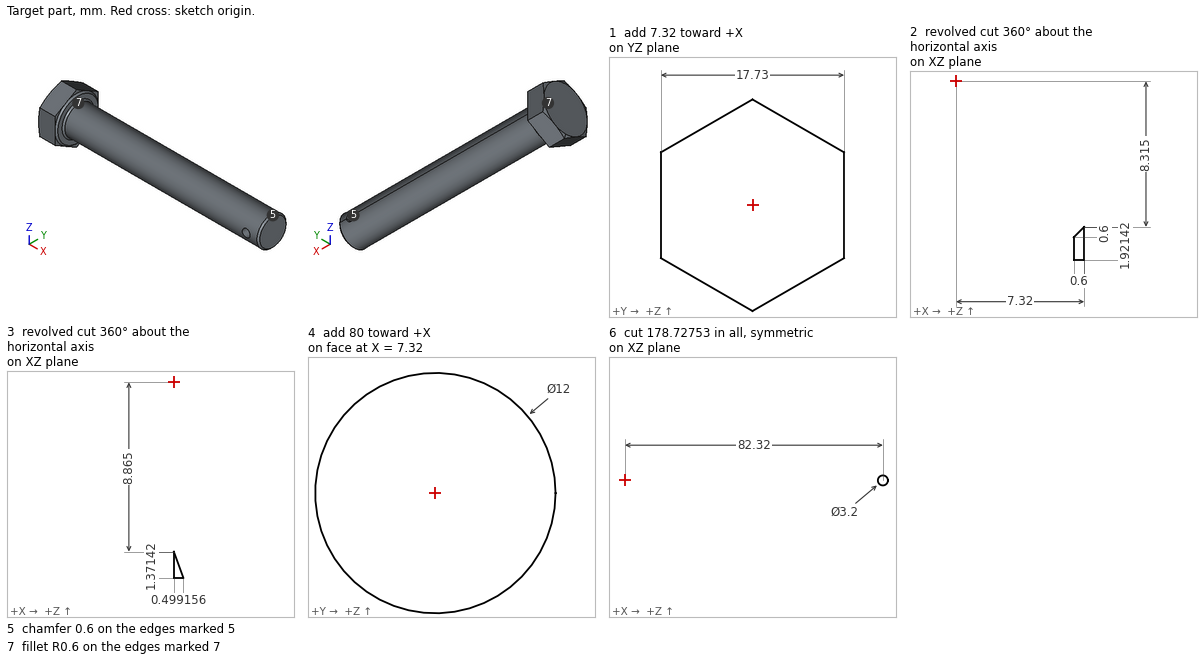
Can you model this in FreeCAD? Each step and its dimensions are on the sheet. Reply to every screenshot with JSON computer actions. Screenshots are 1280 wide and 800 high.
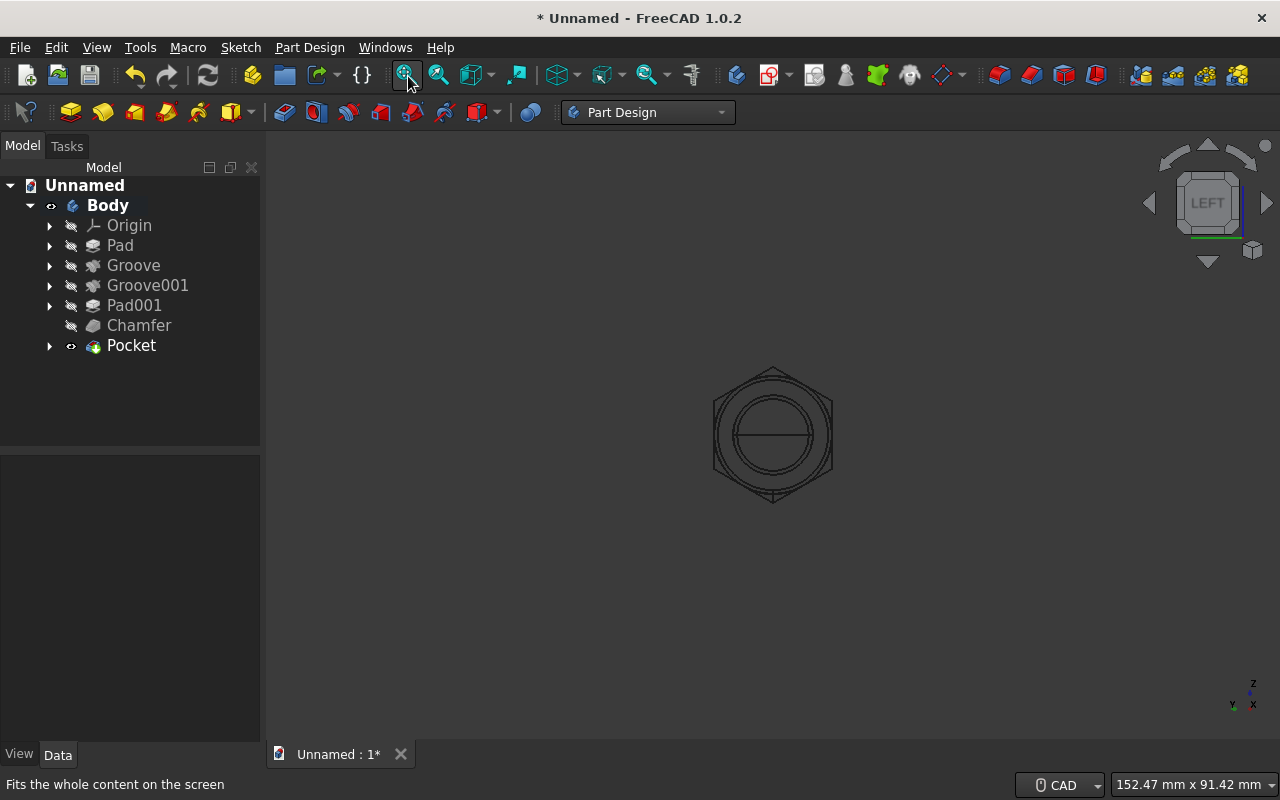
{"action": "key", "text": "0"}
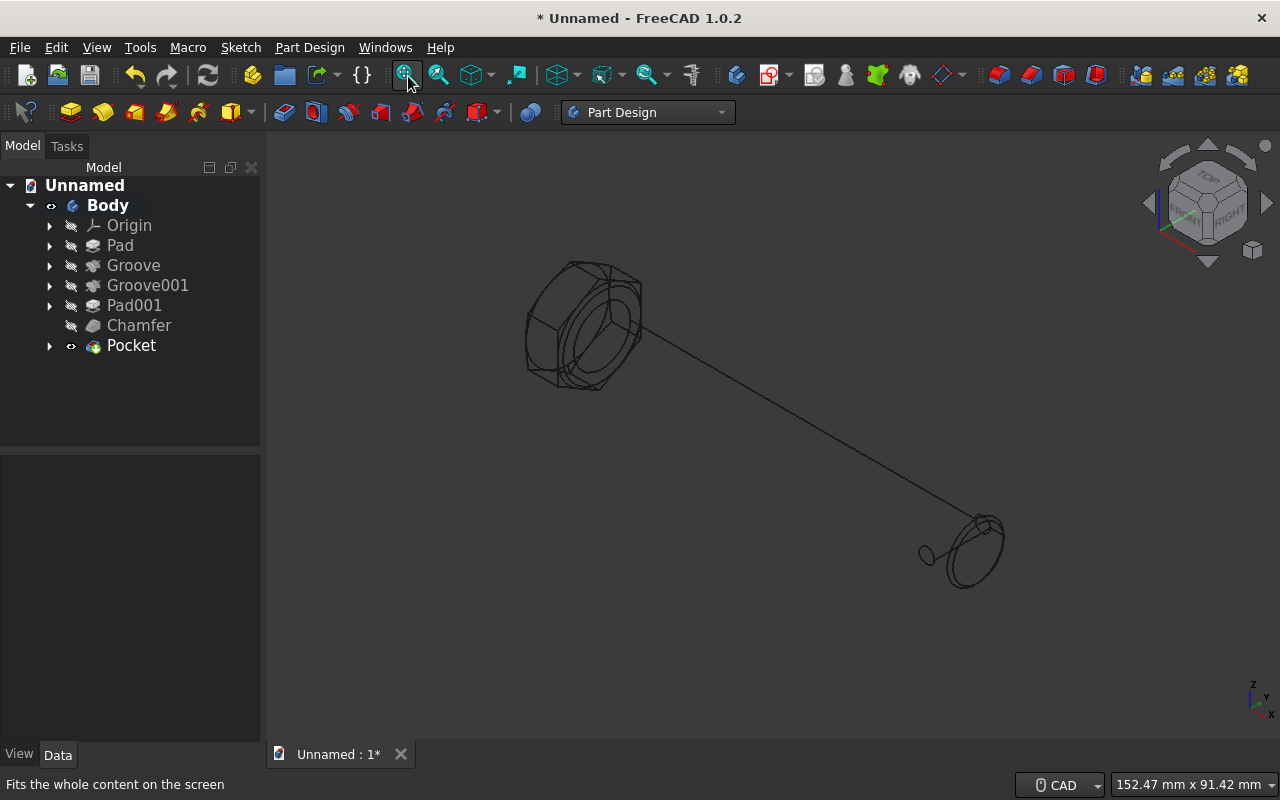
{"action": "left_click", "coordinate": [574, 352]}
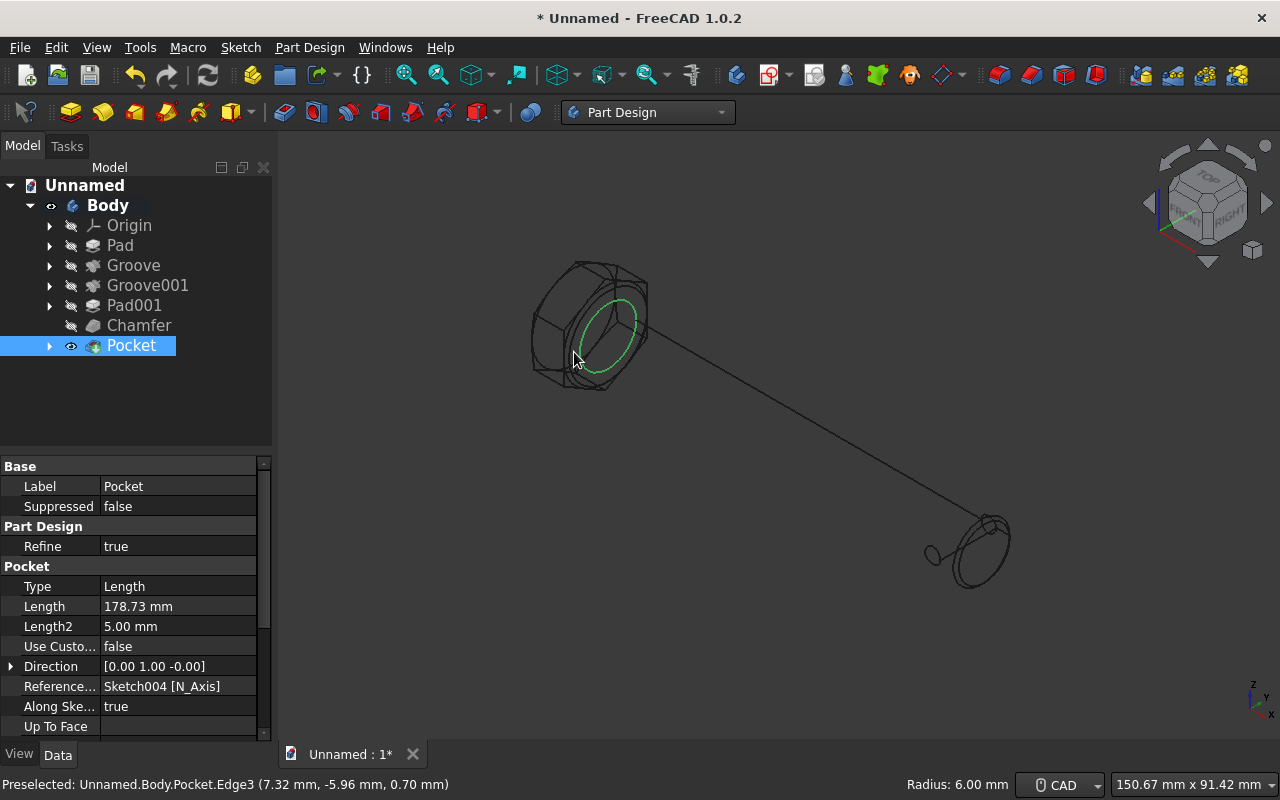
{"action": "key", "text": "v 1"}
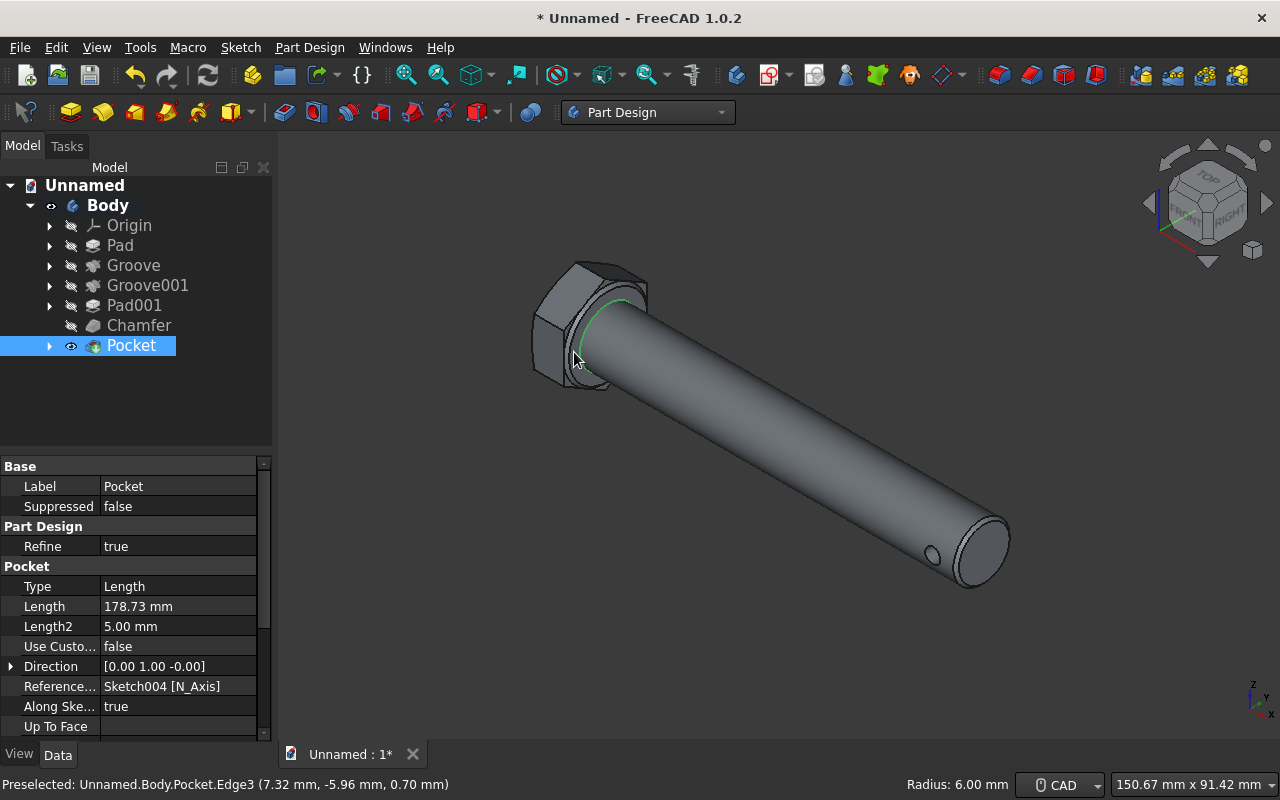
{"action": "left_click", "coordinate": [1000, 76]}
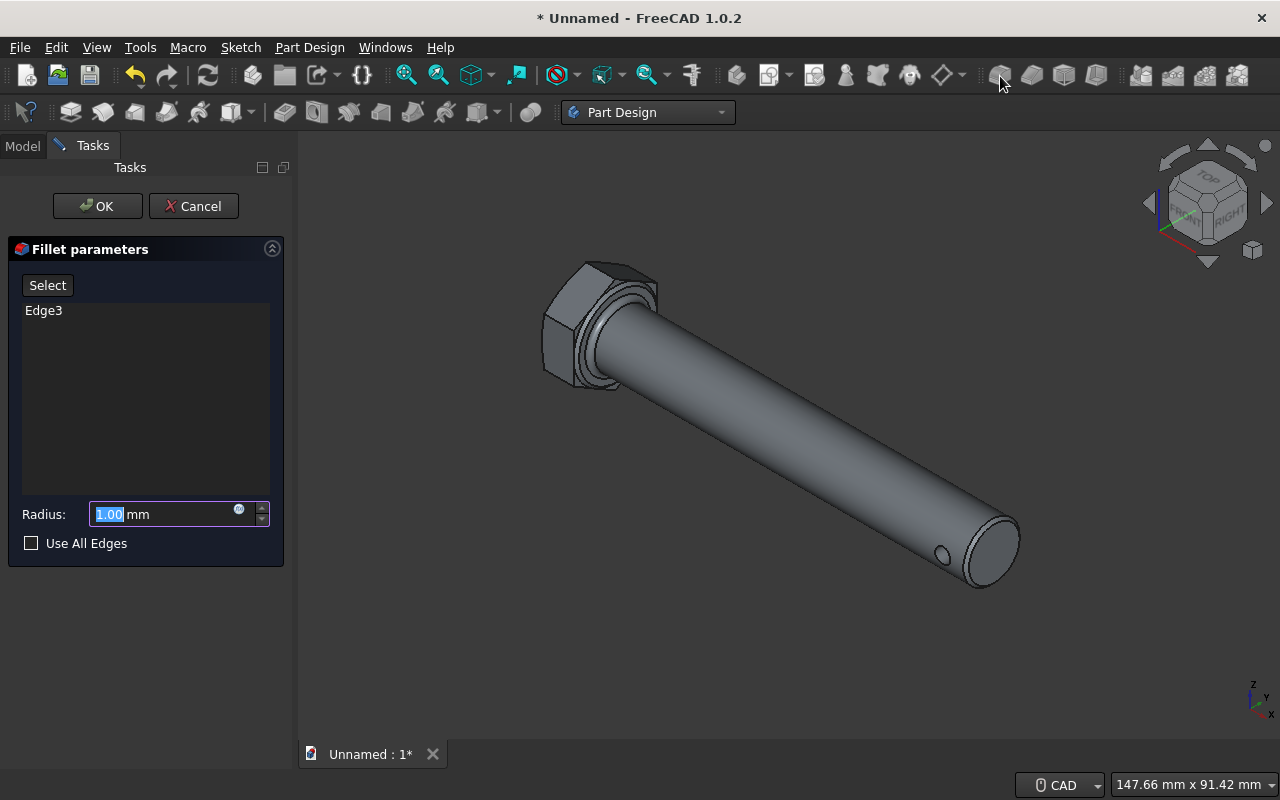
{"action": "type", "text": "0.6"}
{"action": "key", "text": "Tab"}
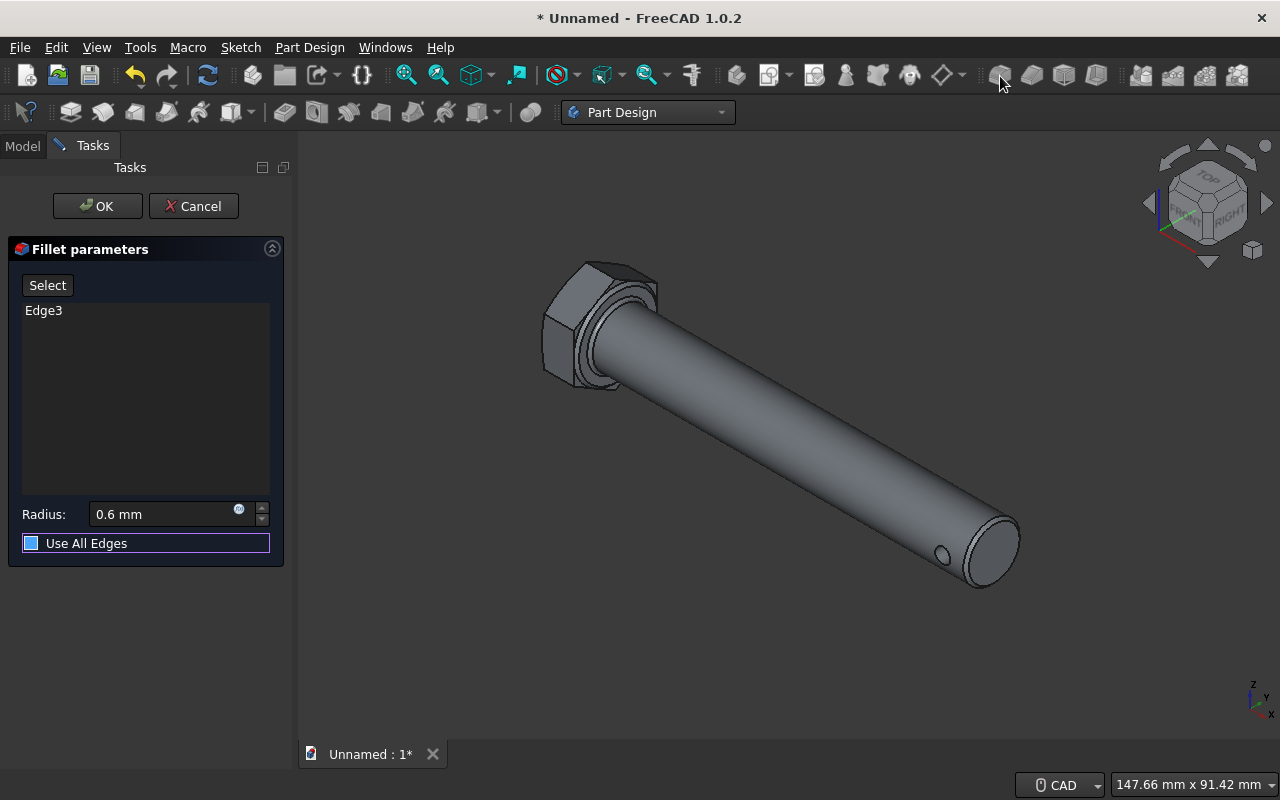
{"action": "left_click", "coordinate": [98, 206]}